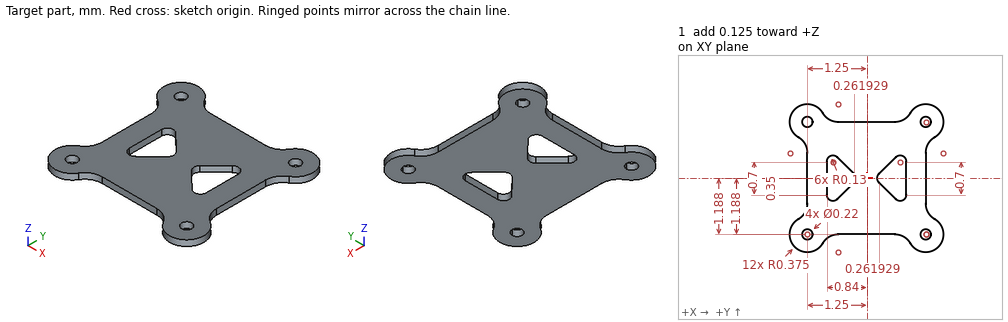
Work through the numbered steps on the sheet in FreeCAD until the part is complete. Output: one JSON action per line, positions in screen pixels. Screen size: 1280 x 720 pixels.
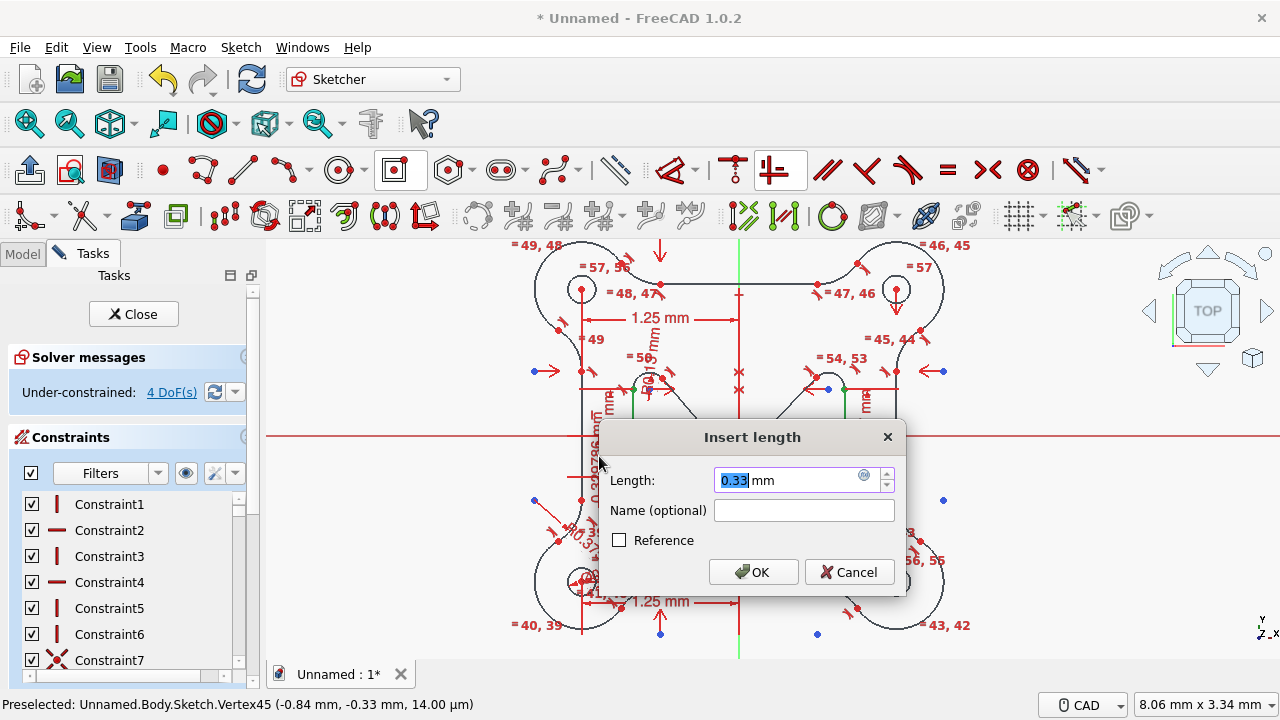
{"action": "type", "text": "0.35"}
{"action": "key", "text": "Return"}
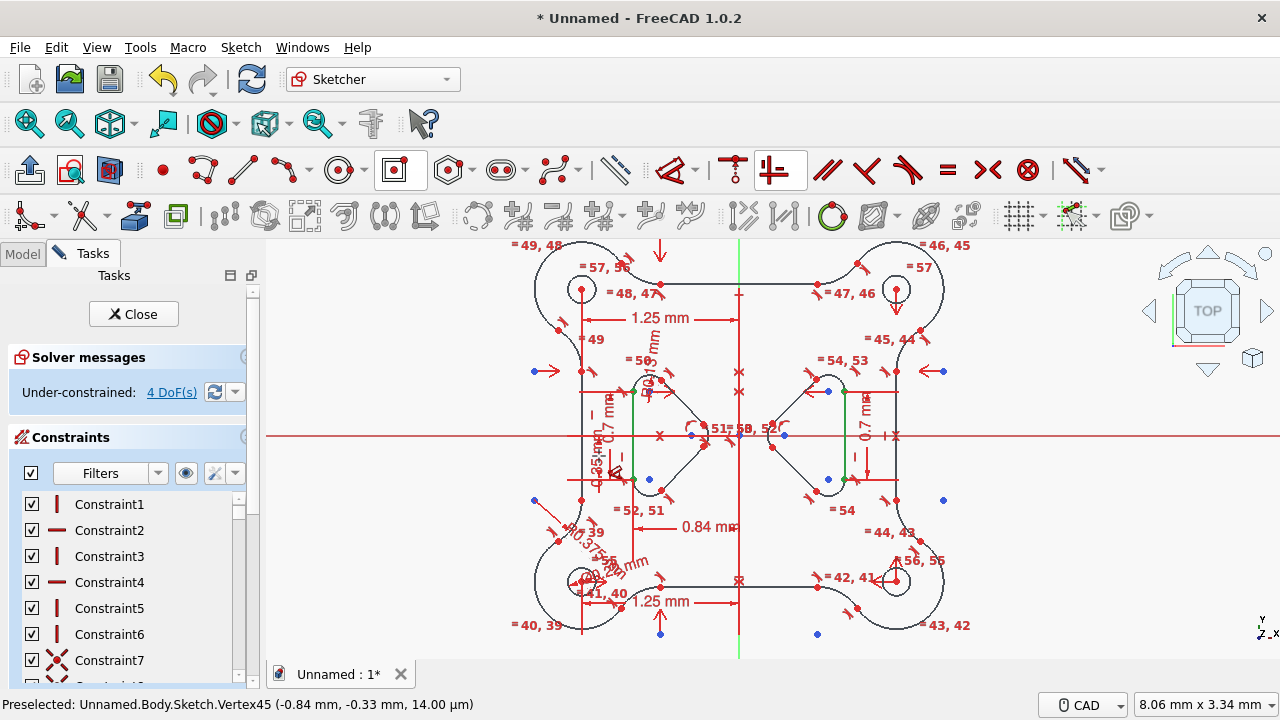
{"action": "left_click", "coordinate": [582, 582]}
{"action": "left_click", "coordinate": [548, 509]}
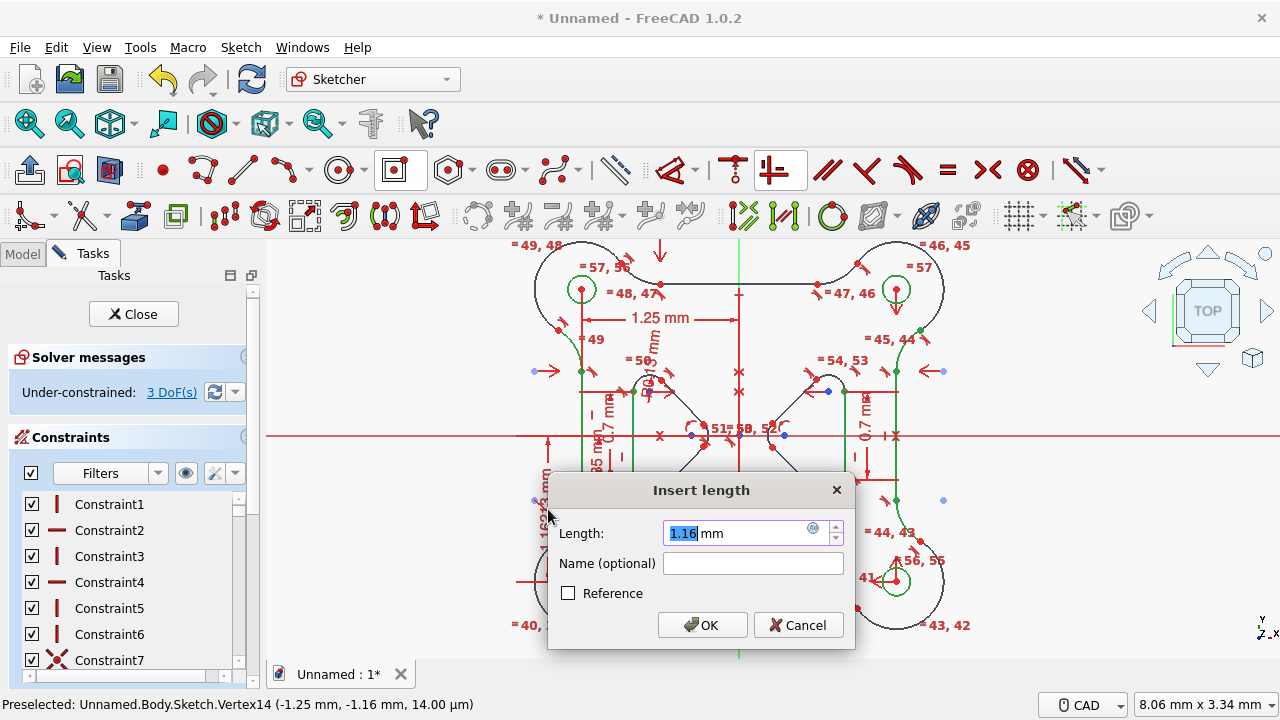
{"action": "type", "text": "1.188"}
{"action": "key", "text": "Return"}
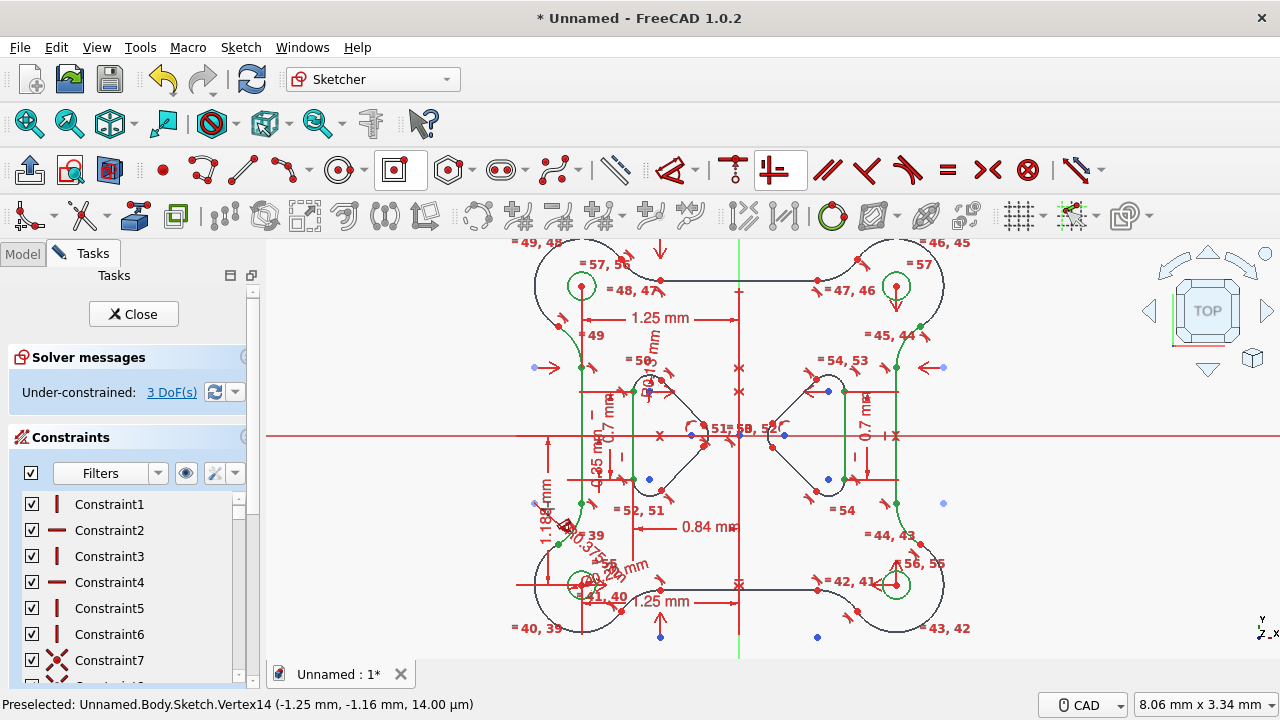
{"action": "left_click", "coordinate": [660, 590]}
{"action": "left_click", "coordinate": [626, 513]}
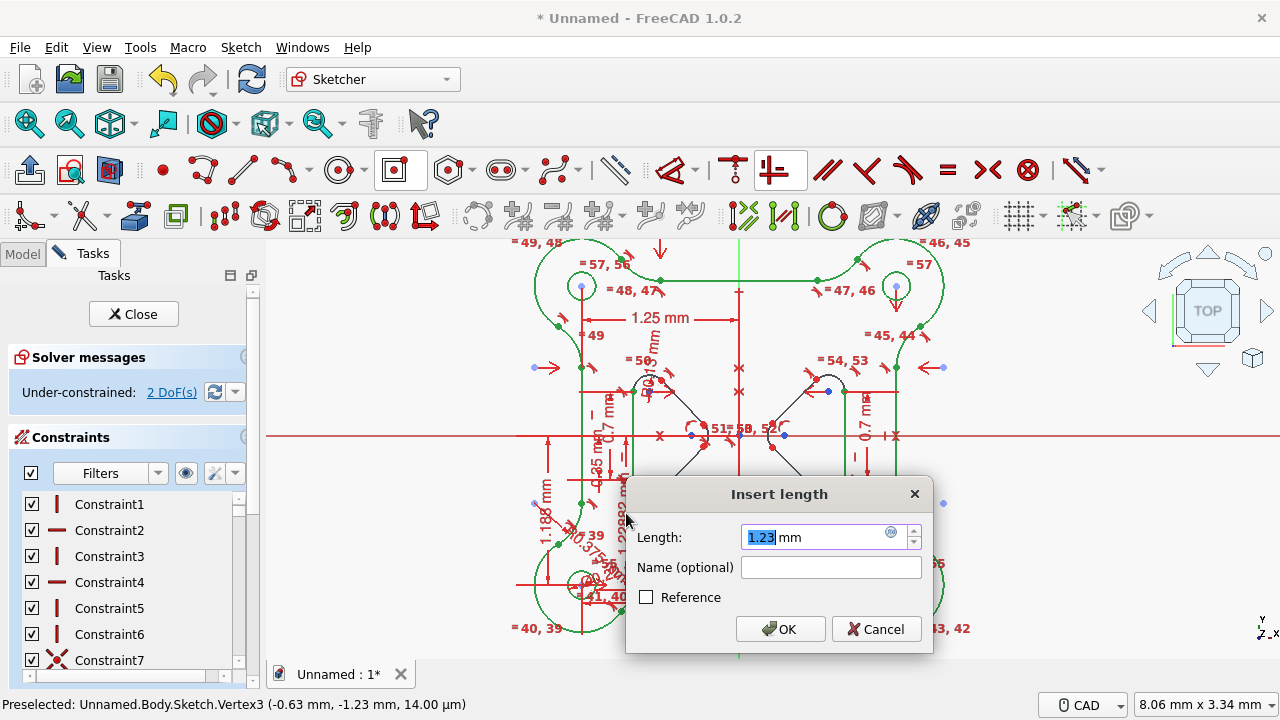
{"action": "type", "text": "1.188"}
{"action": "key", "text": "Return"}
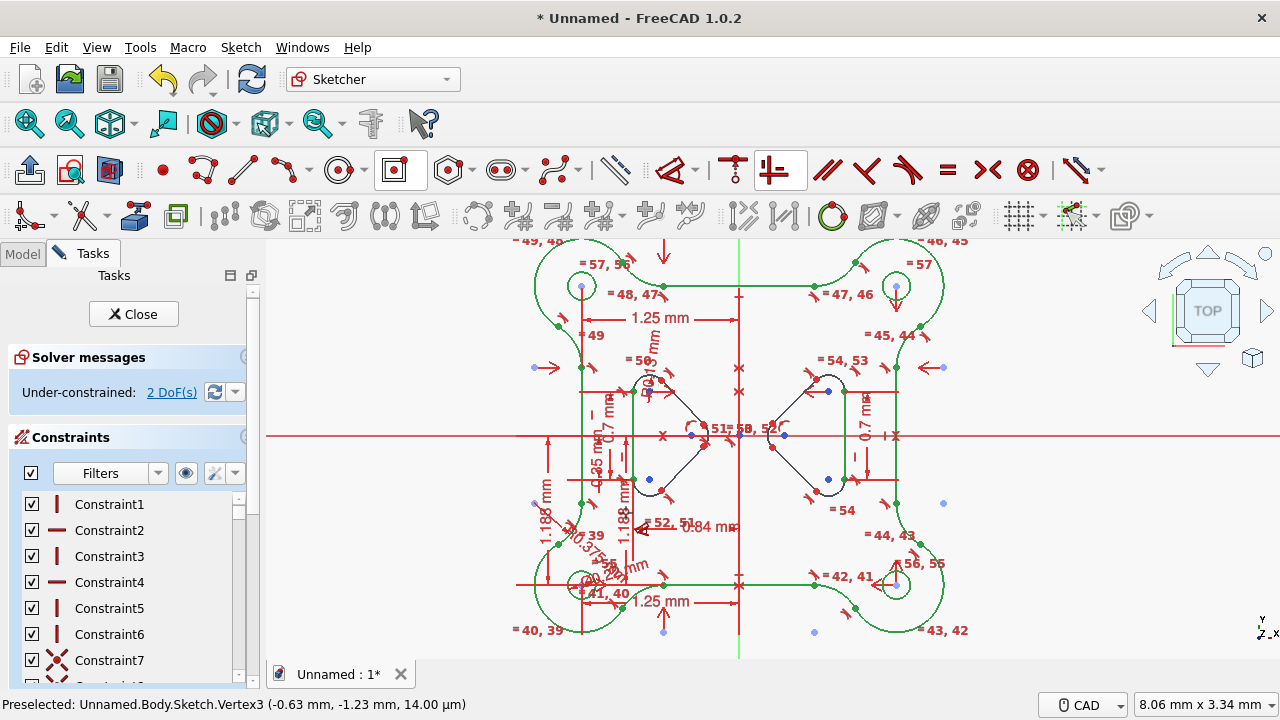
{"action": "left_click", "coordinate": [704, 424]}
{"action": "left_click", "coordinate": [721, 390]}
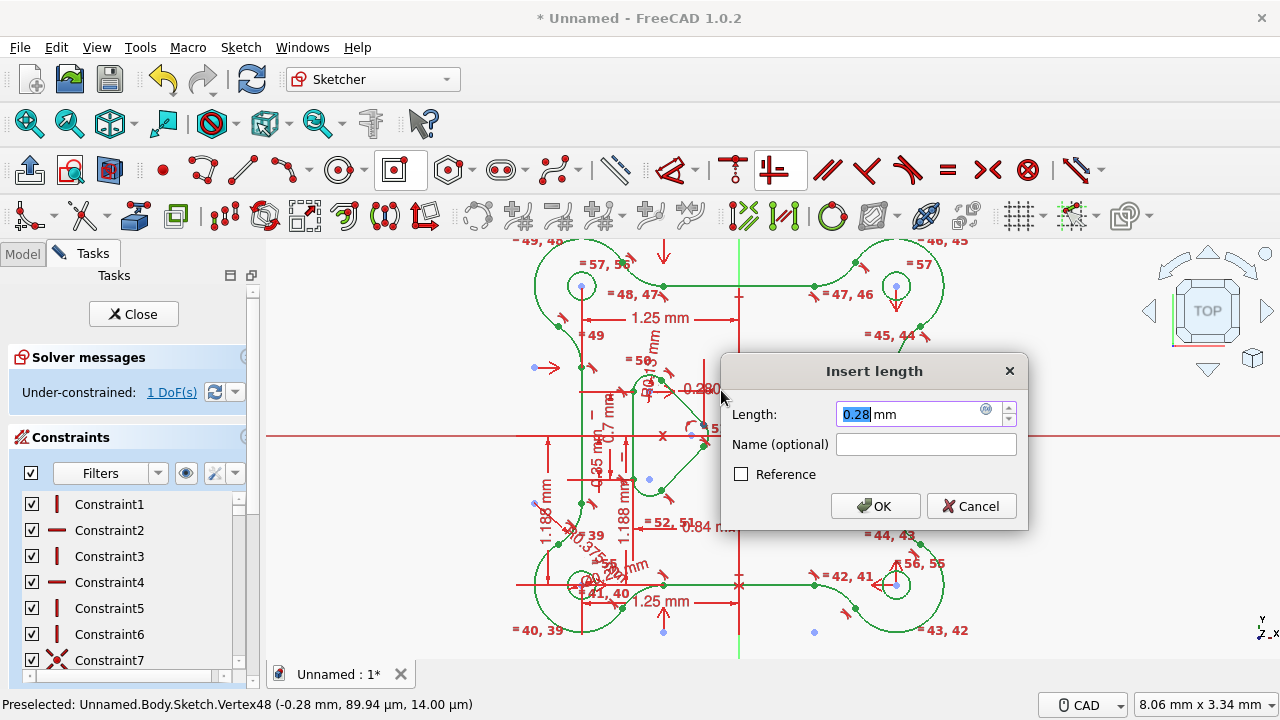
{"action": "type", "text": "0.261929"}
{"action": "key", "text": "Return"}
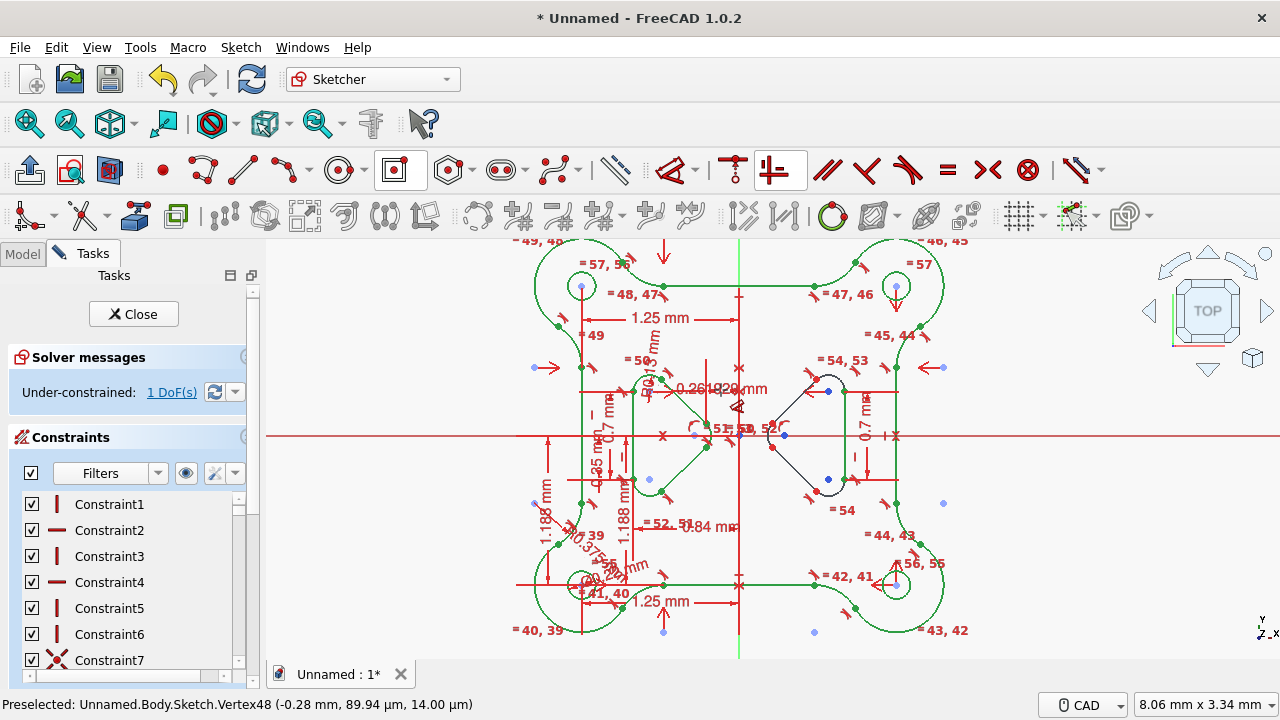
{"action": "left_click", "coordinate": [773, 447]}
{"action": "left_click", "coordinate": [756, 481]}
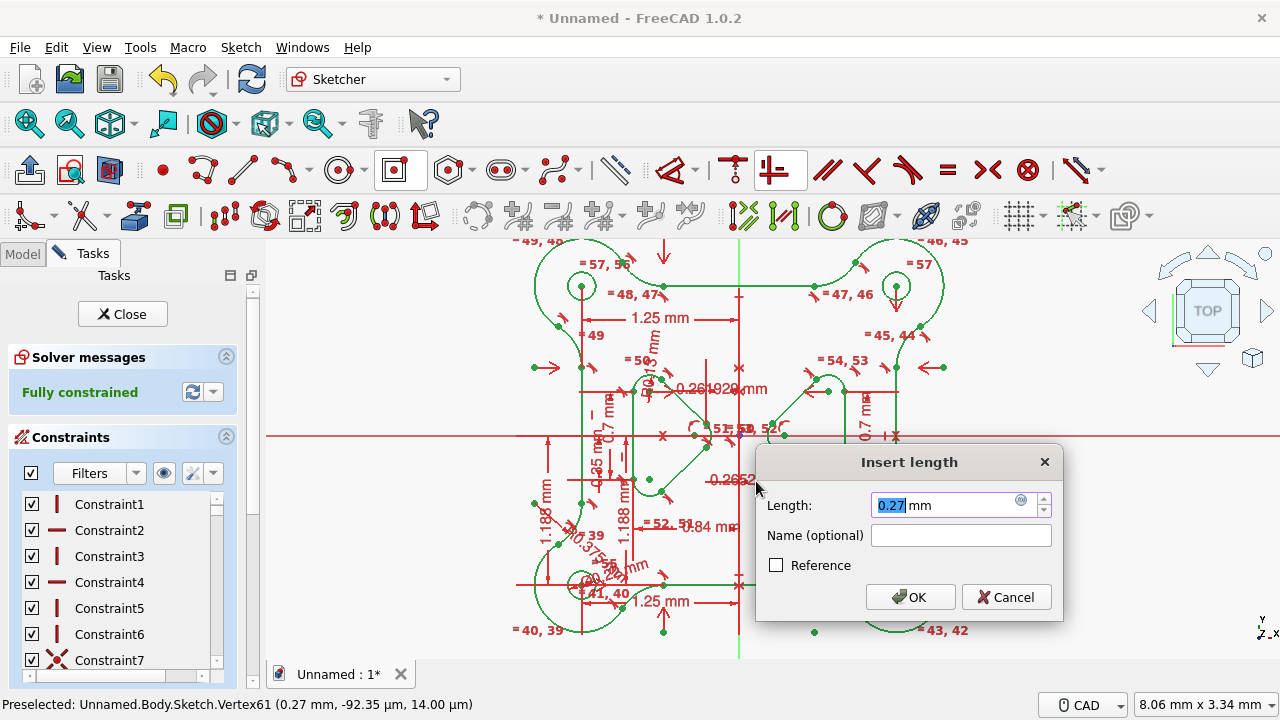
{"action": "type", "text": "0.261929"}
{"action": "key", "text": "Return"}
{"action": "key", "text": "Escape"}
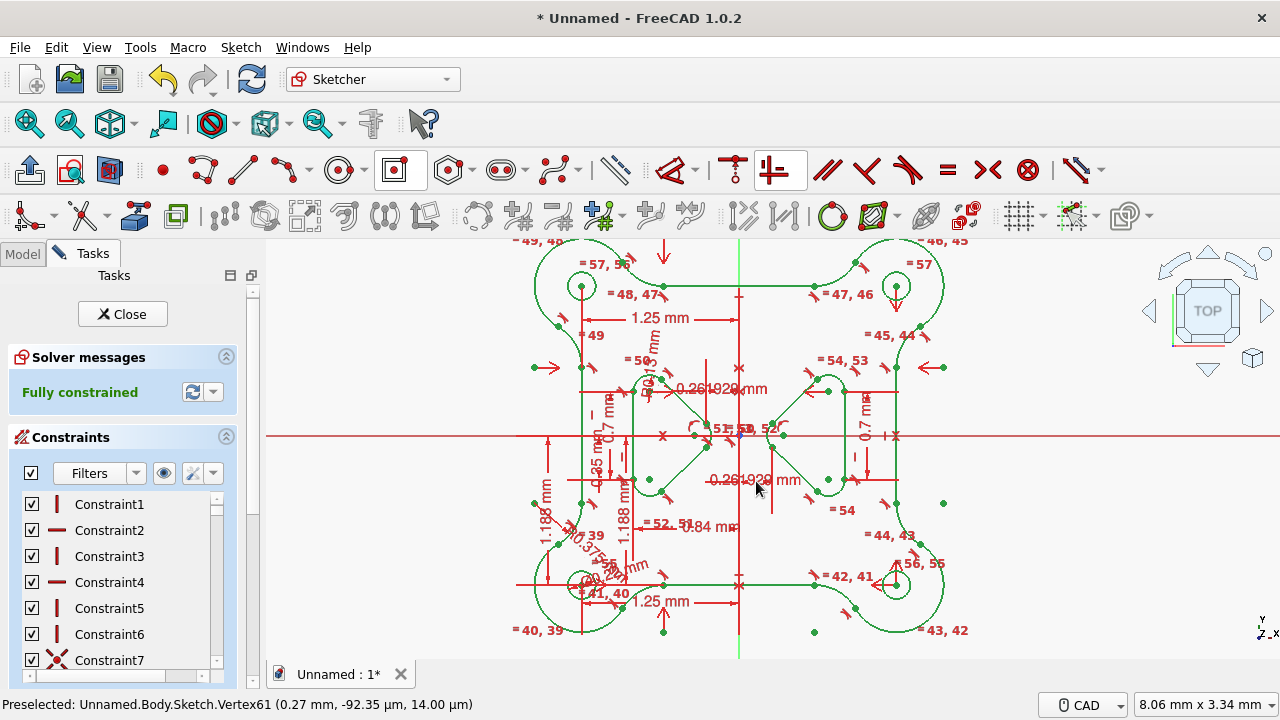
{"action": "left_click", "coordinate": [123, 314]}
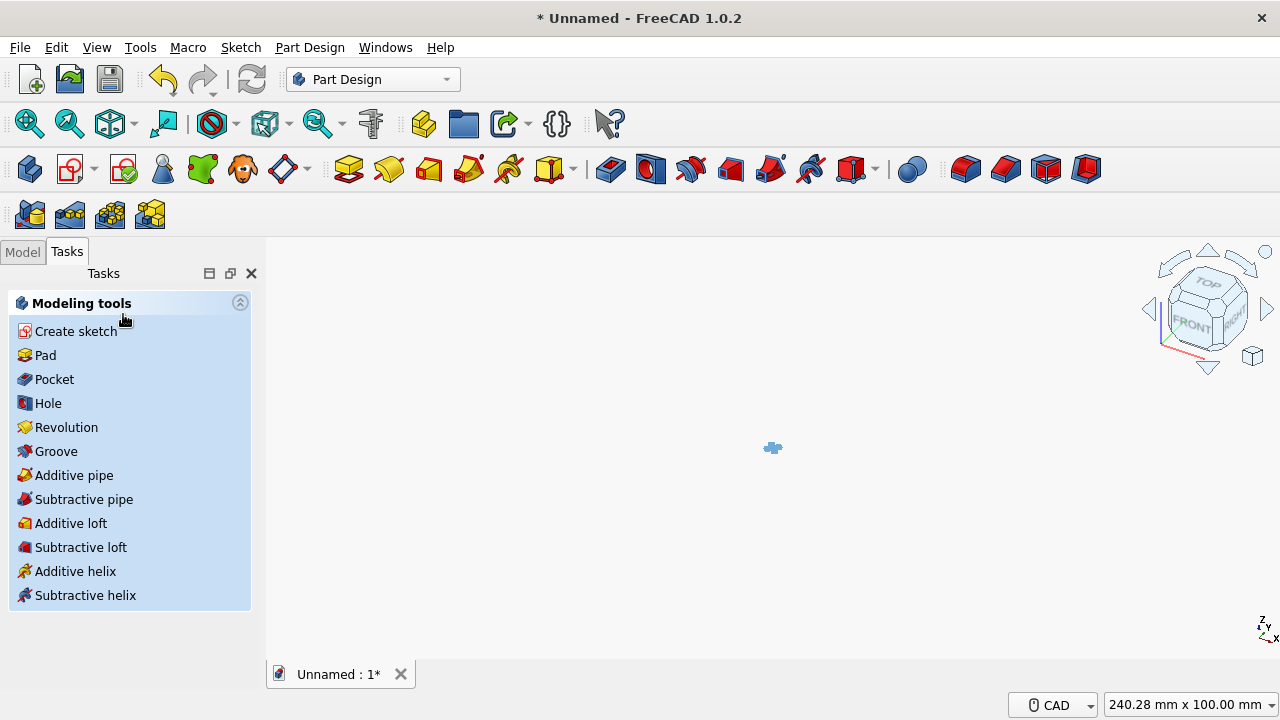
{"action": "left_click", "coordinate": [350, 170]}